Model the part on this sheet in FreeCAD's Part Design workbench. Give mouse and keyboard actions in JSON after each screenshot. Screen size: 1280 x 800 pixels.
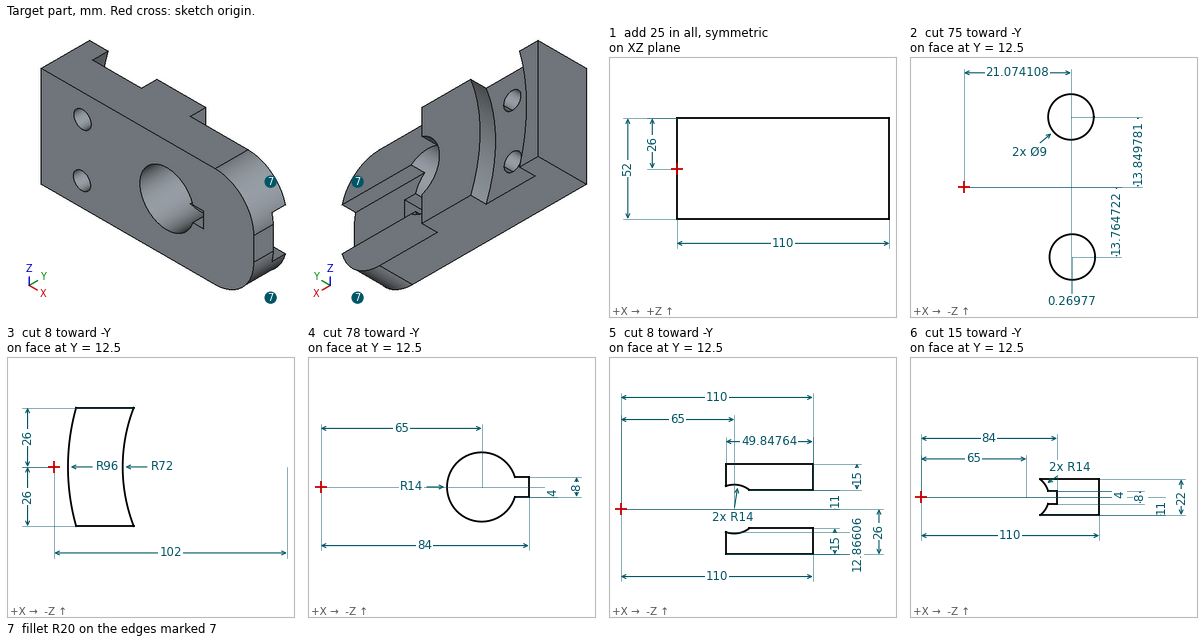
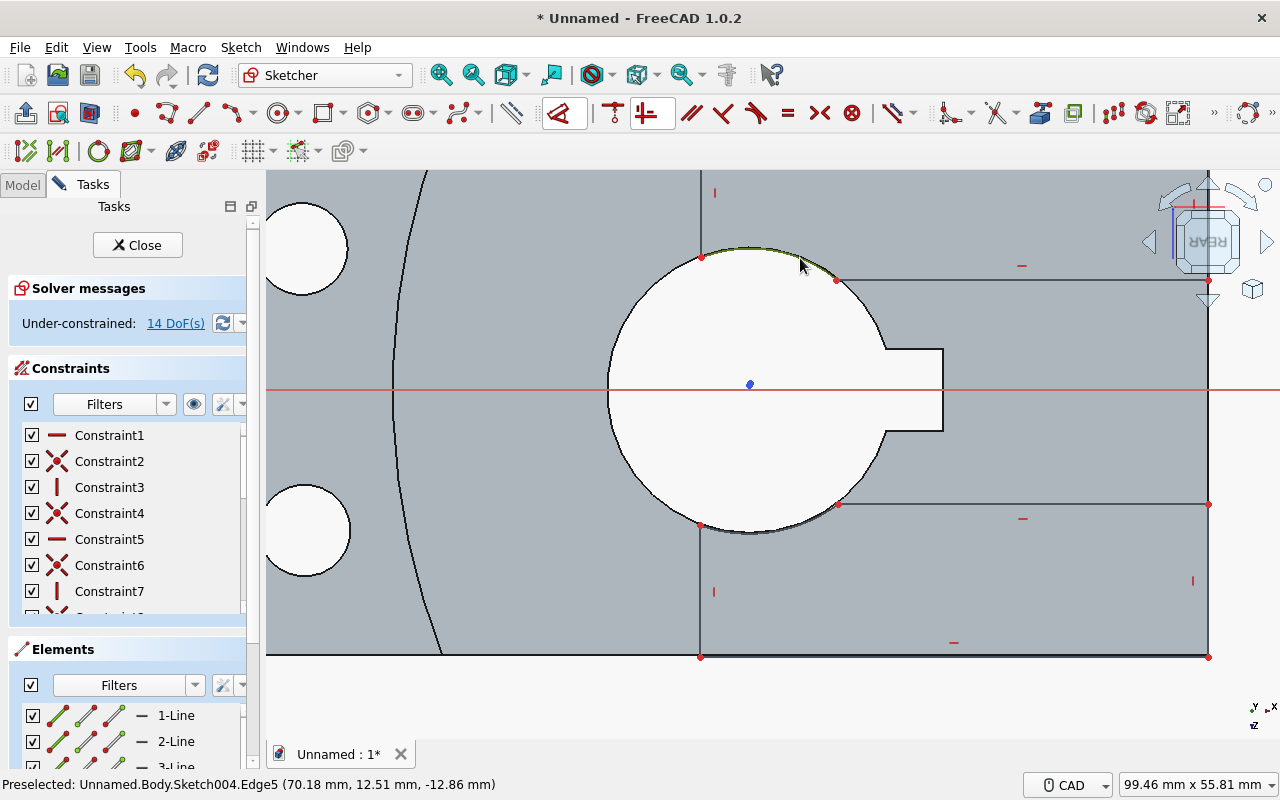
{"action": "left_click", "coordinate": [743, 534]}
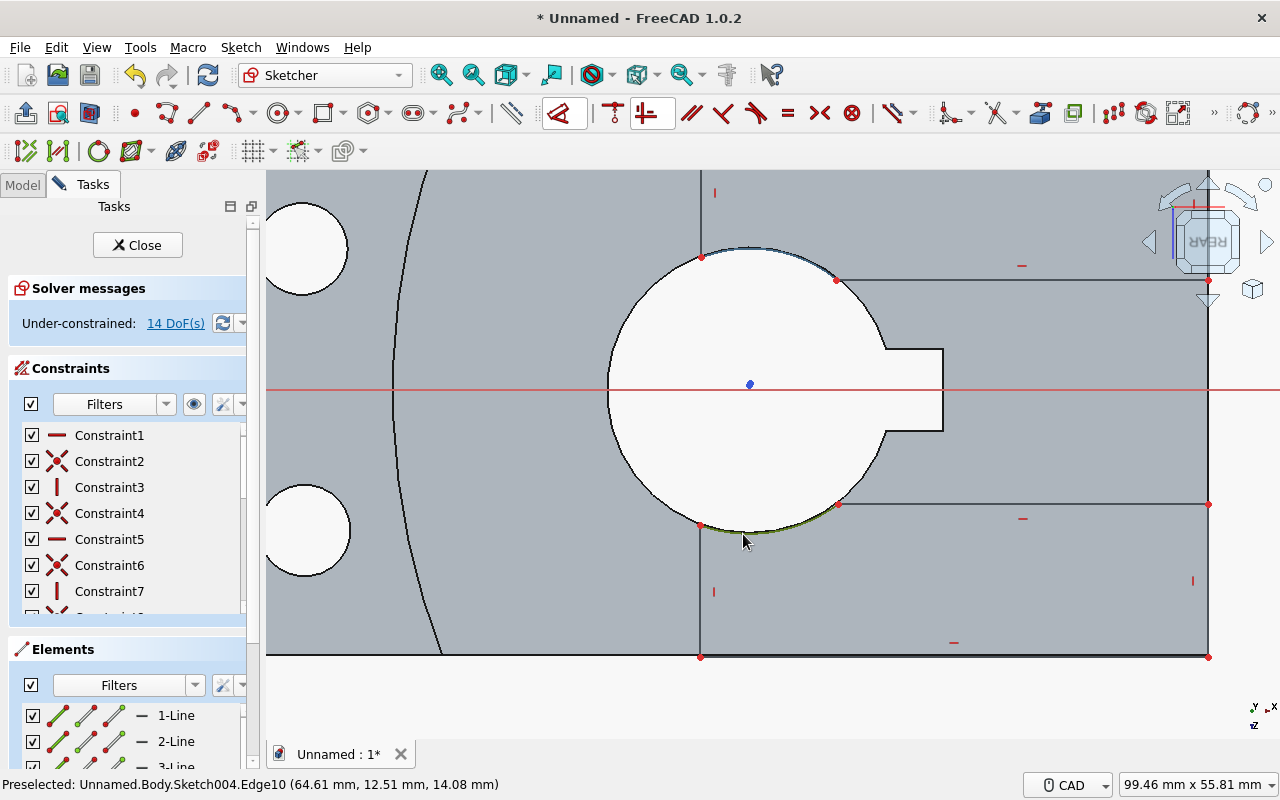
{"action": "left_click", "coordinate": [614, 114]}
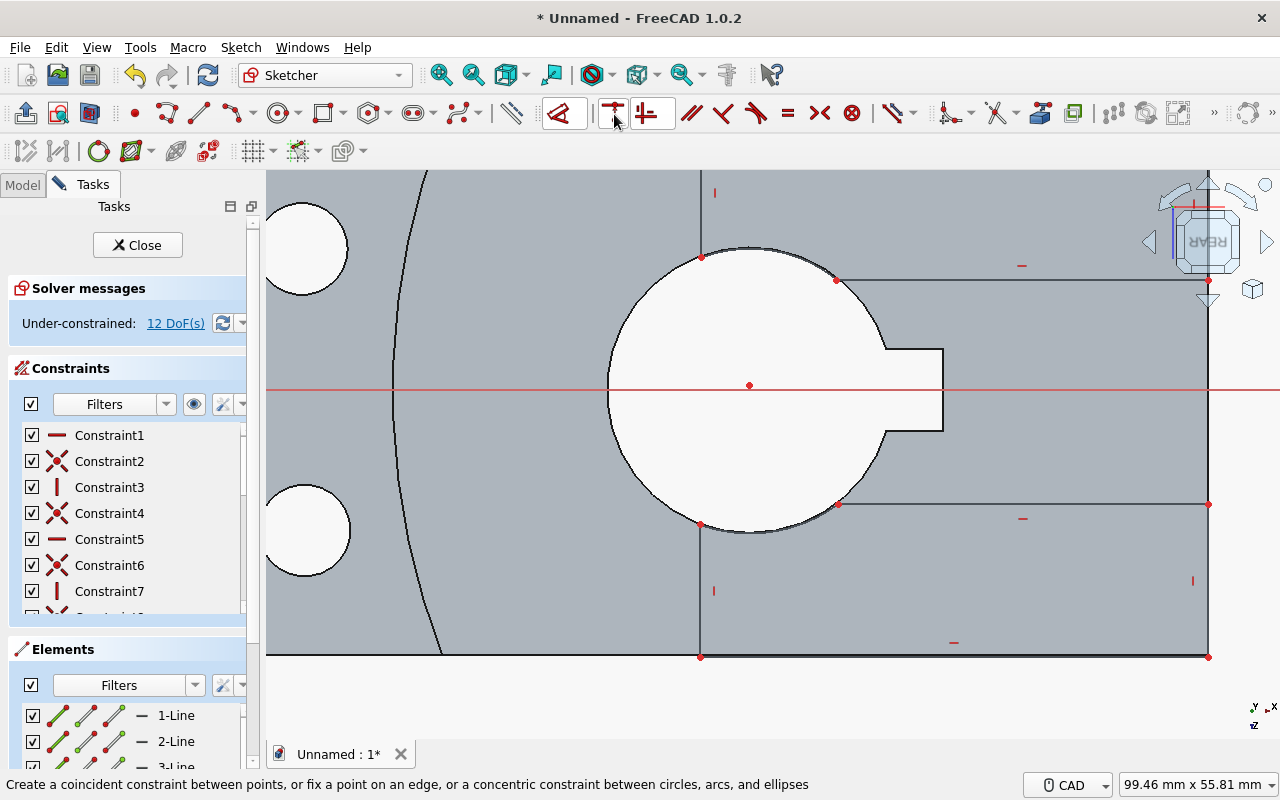
{"action": "left_click", "coordinate": [800, 258]}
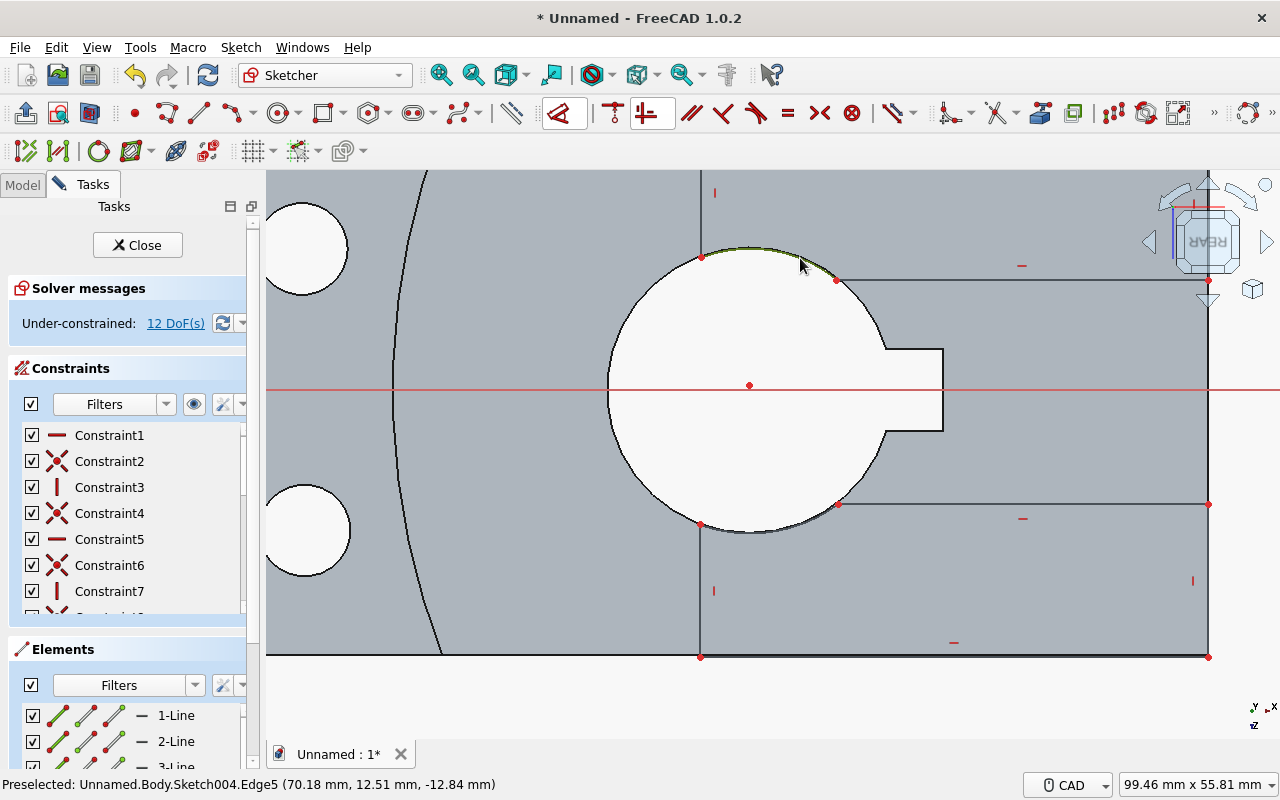
{"action": "left_click", "coordinate": [743, 533]}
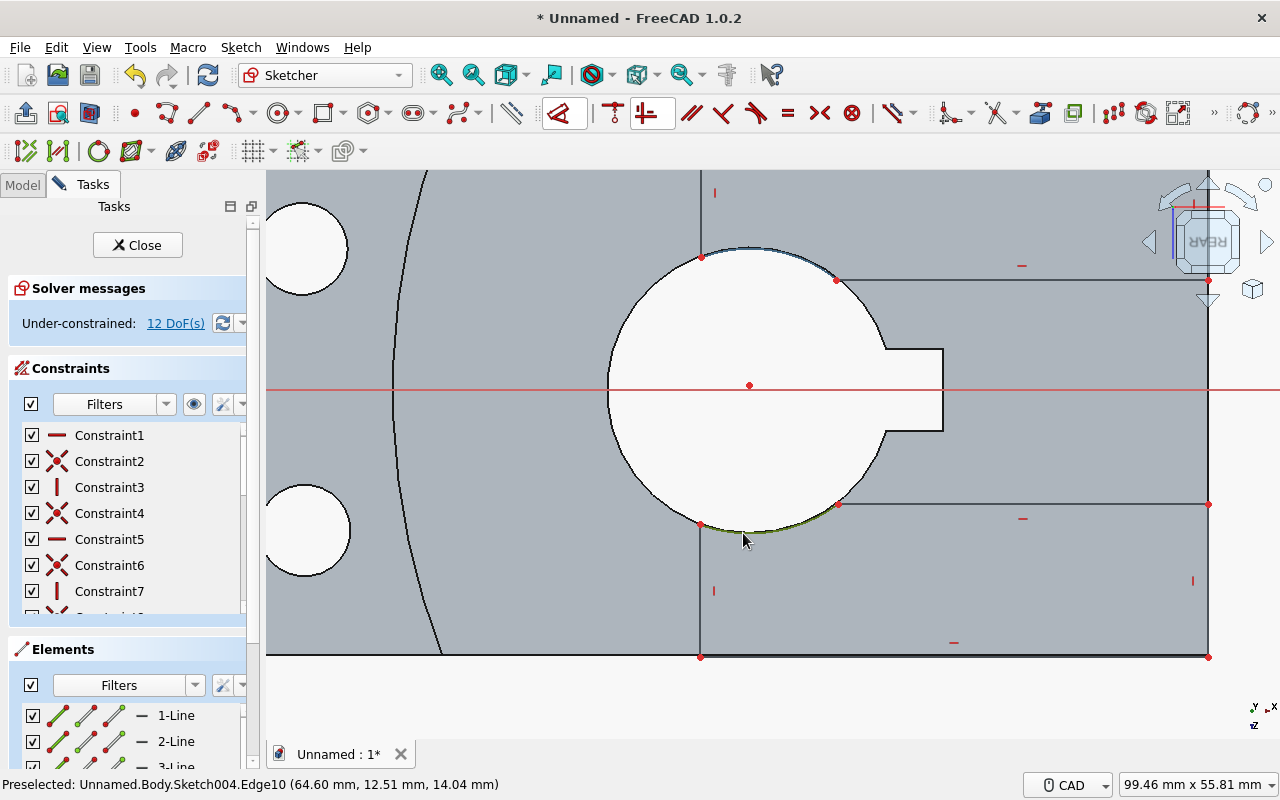
{"action": "left_click", "coordinate": [788, 114]}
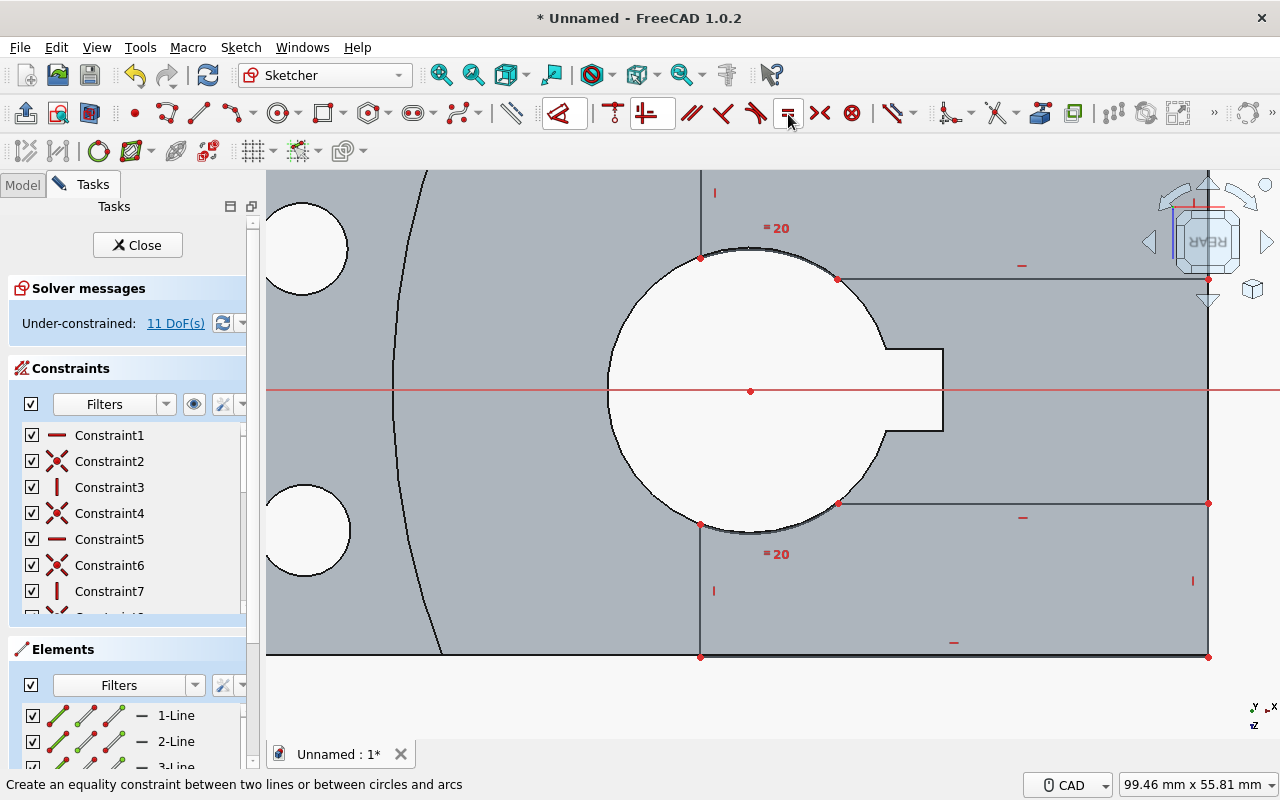
{"action": "left_click", "coordinate": [750, 392]}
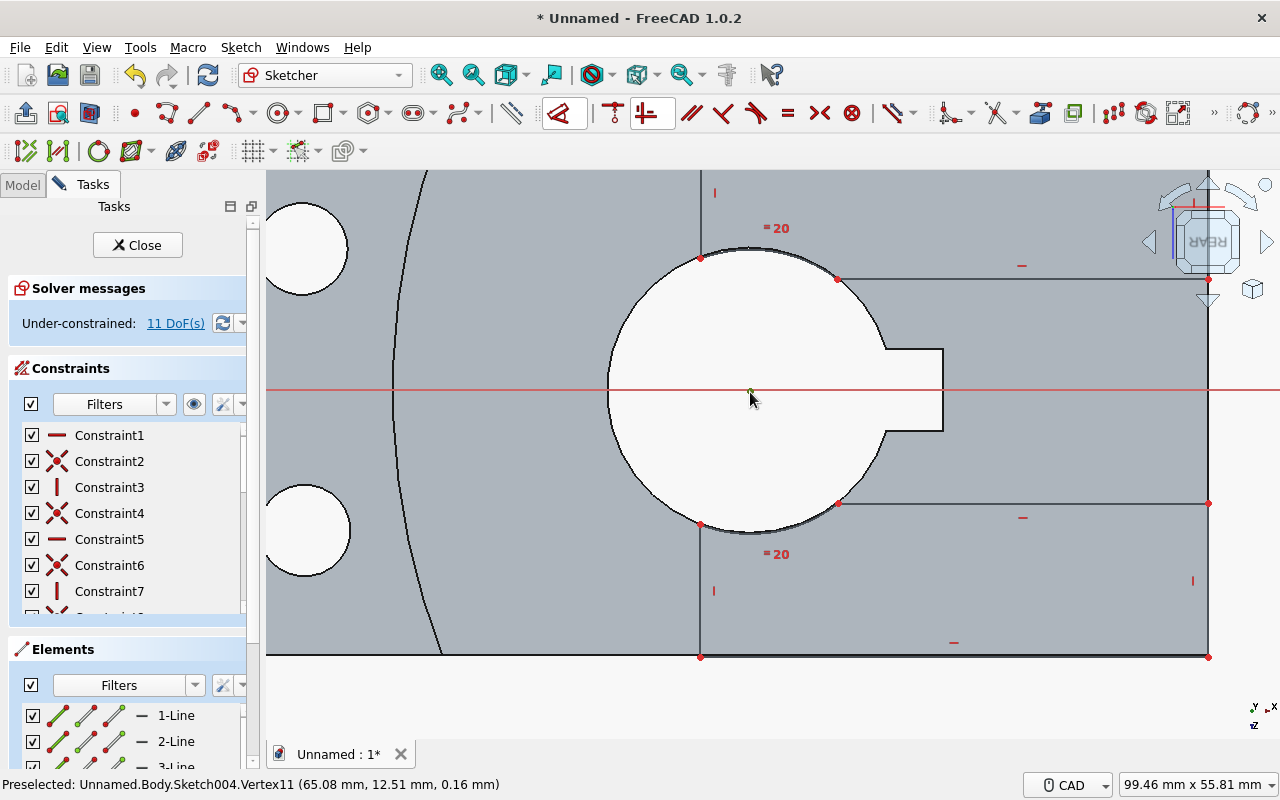
{"action": "left_click", "coordinate": [353, 390]}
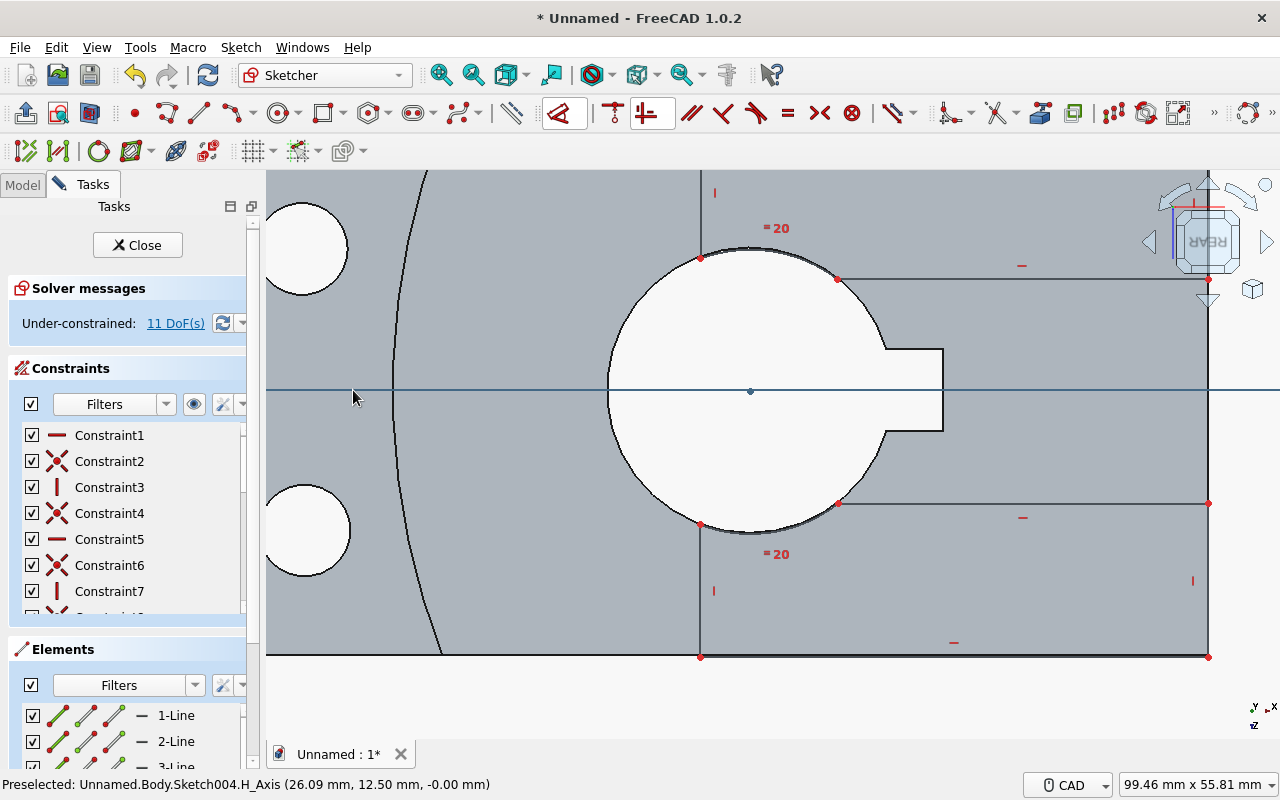
{"action": "left_click", "coordinate": [614, 114]}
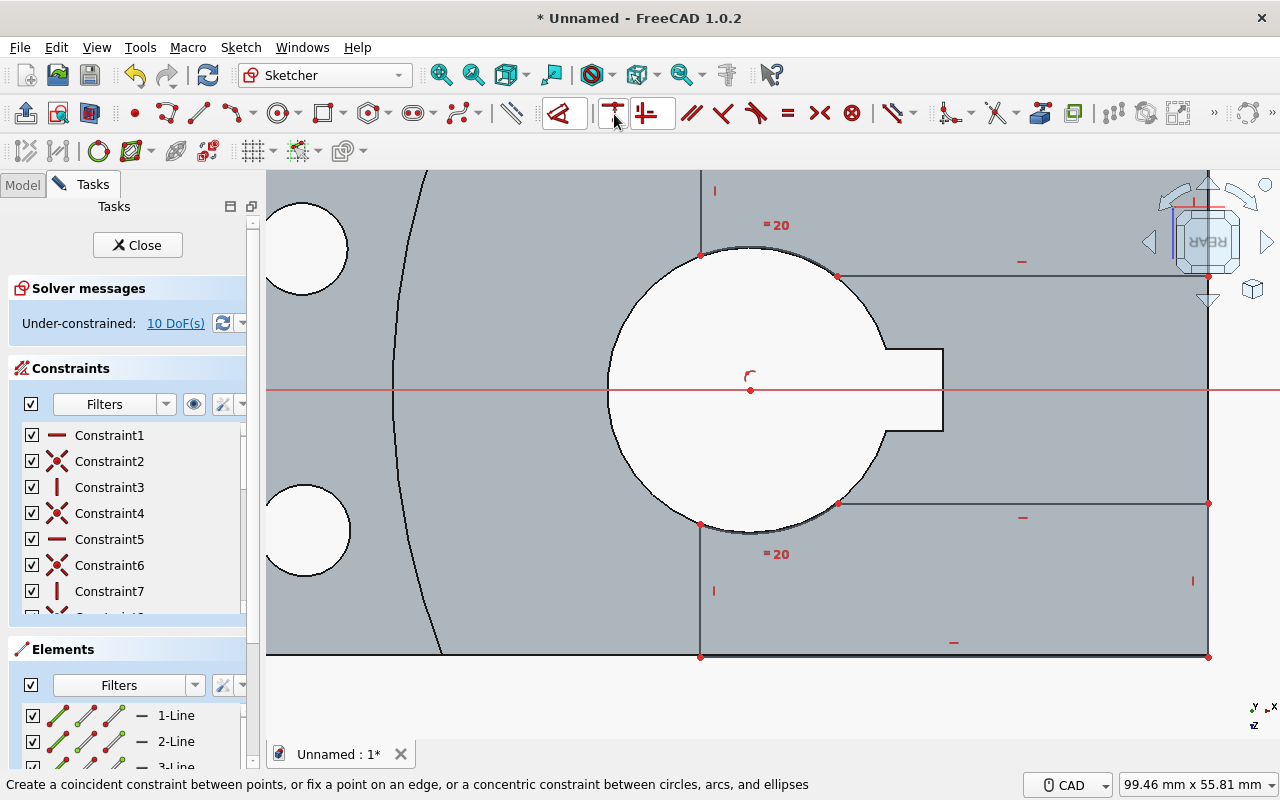
{"action": "left_click", "coordinate": [800, 255]}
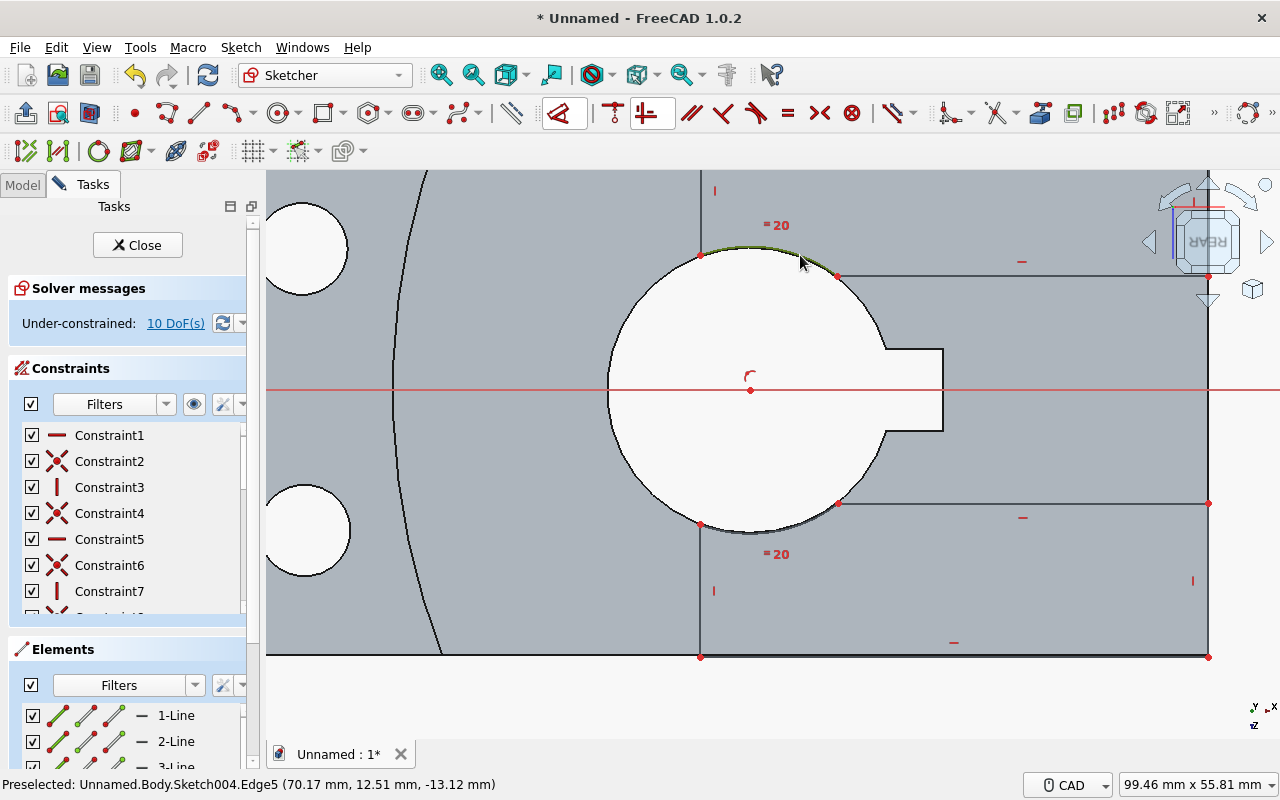
{"action": "key", "text": "k r"}